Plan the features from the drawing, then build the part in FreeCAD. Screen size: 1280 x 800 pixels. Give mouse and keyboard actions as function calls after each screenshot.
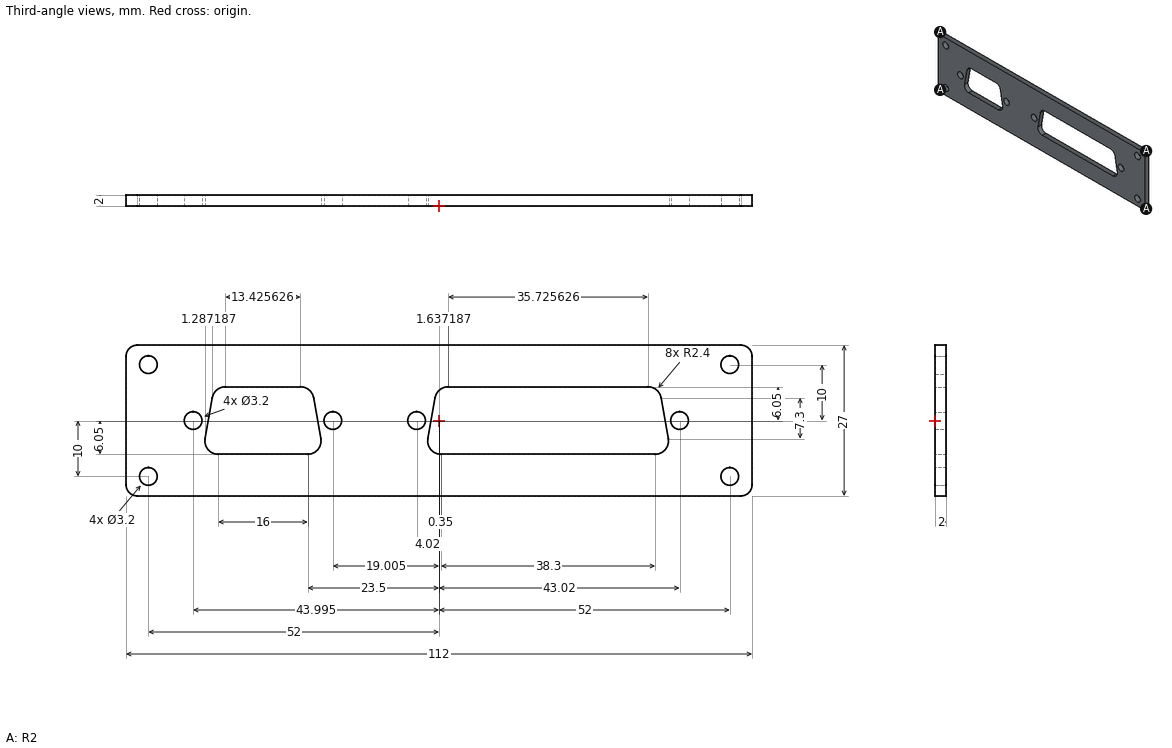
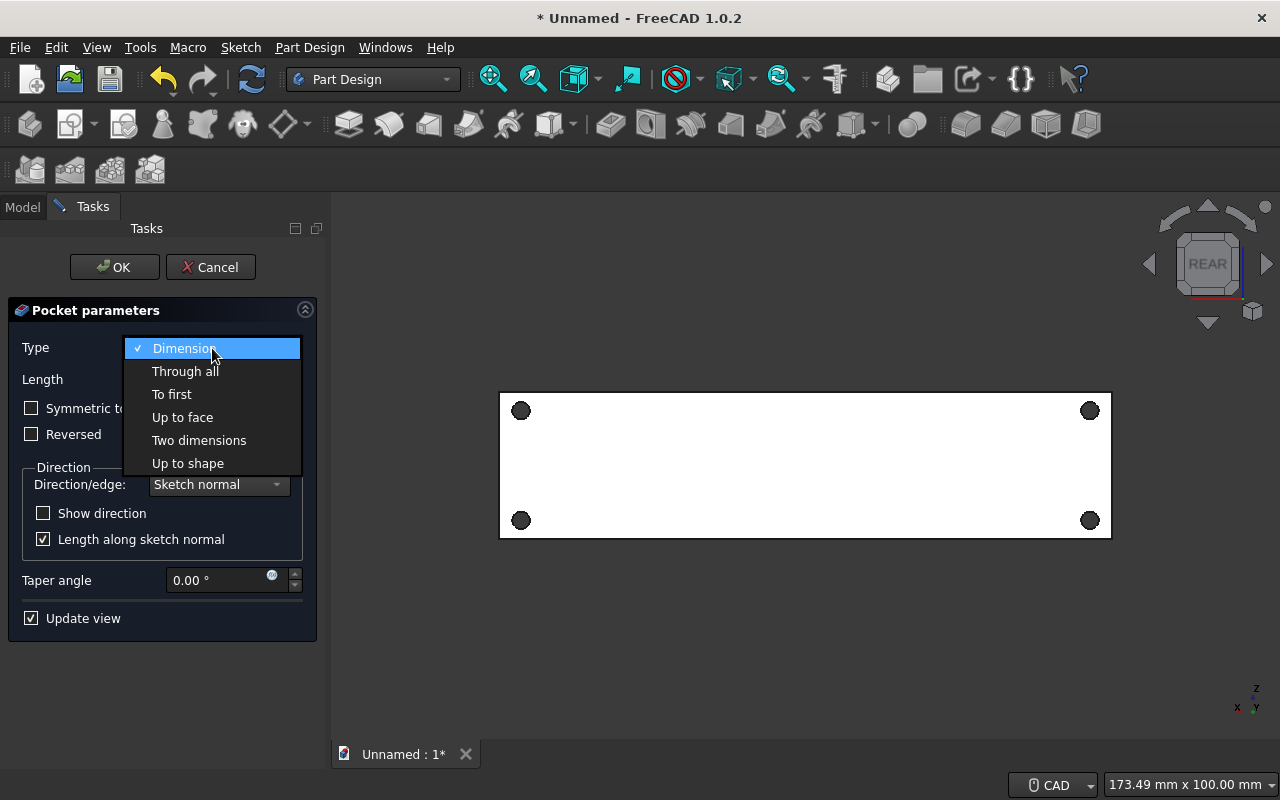
click(212, 372)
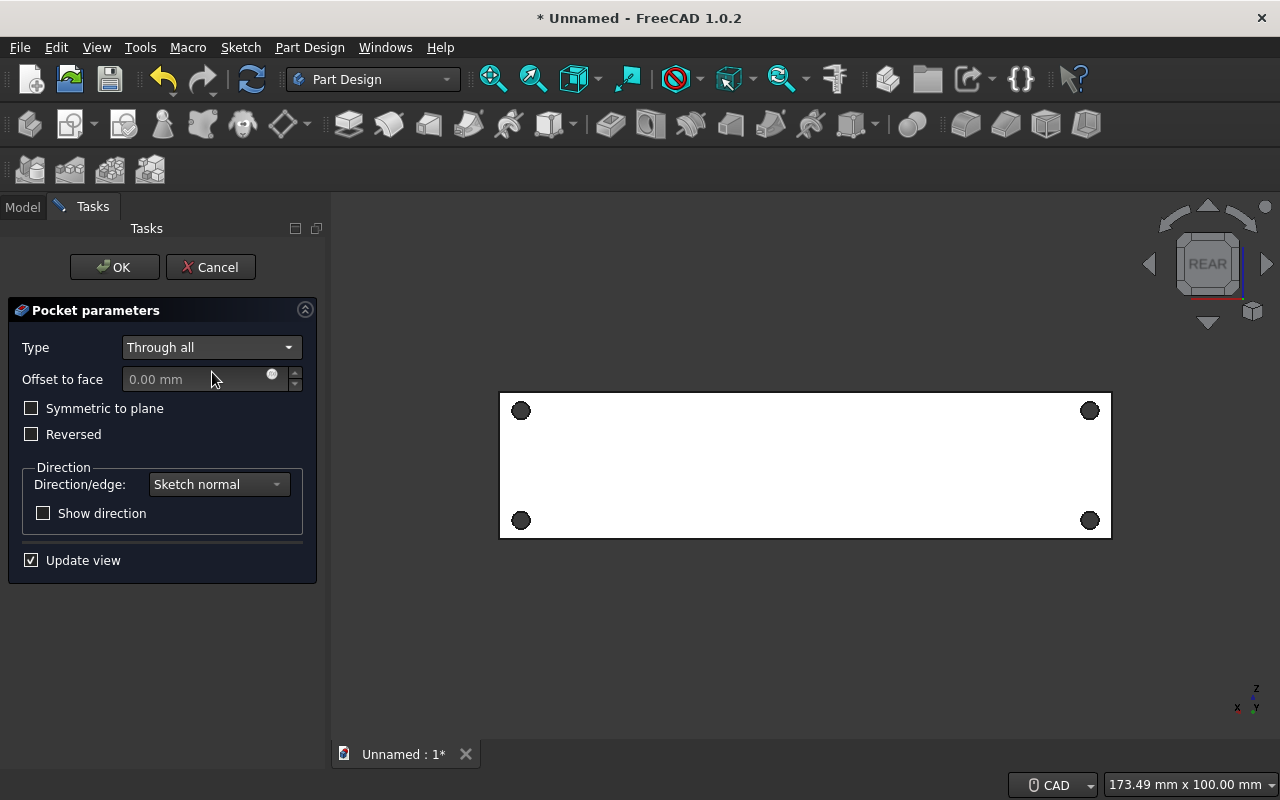
click(115, 267)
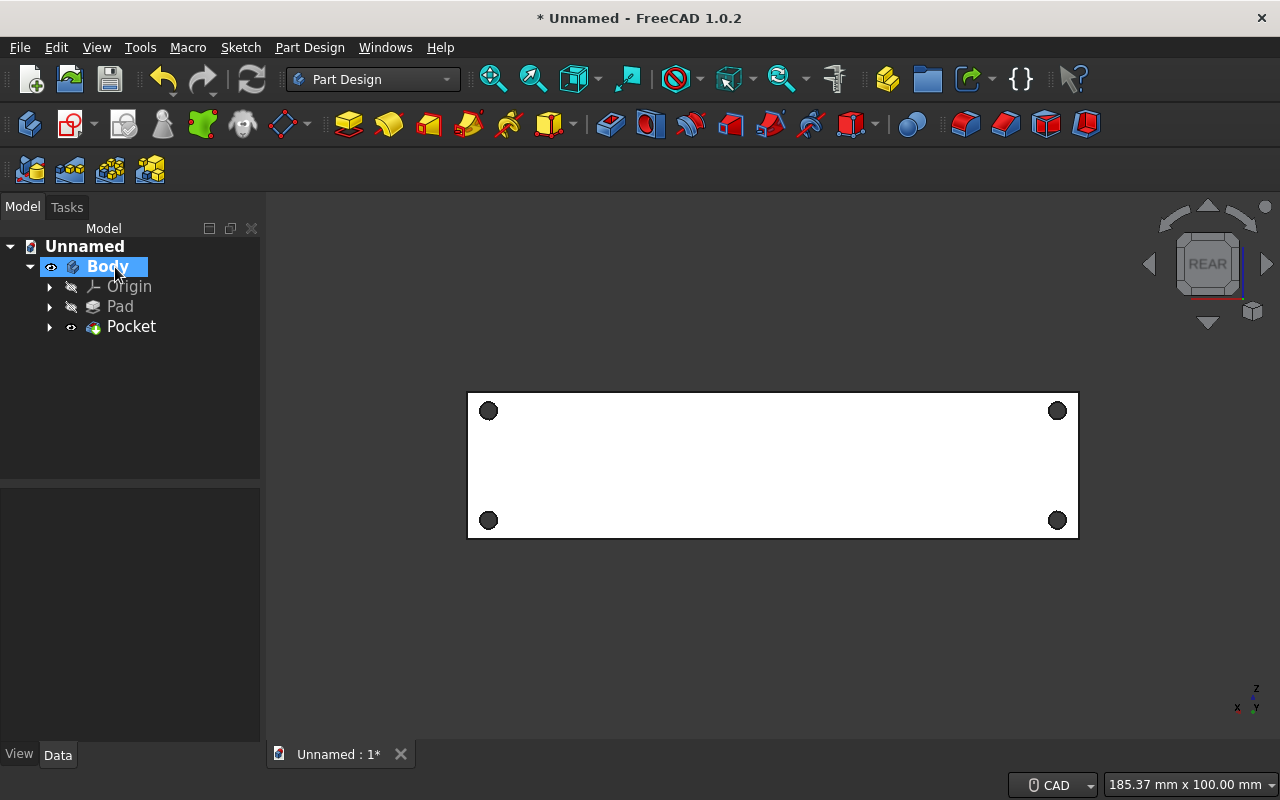
scroll(467, 391, up, 7)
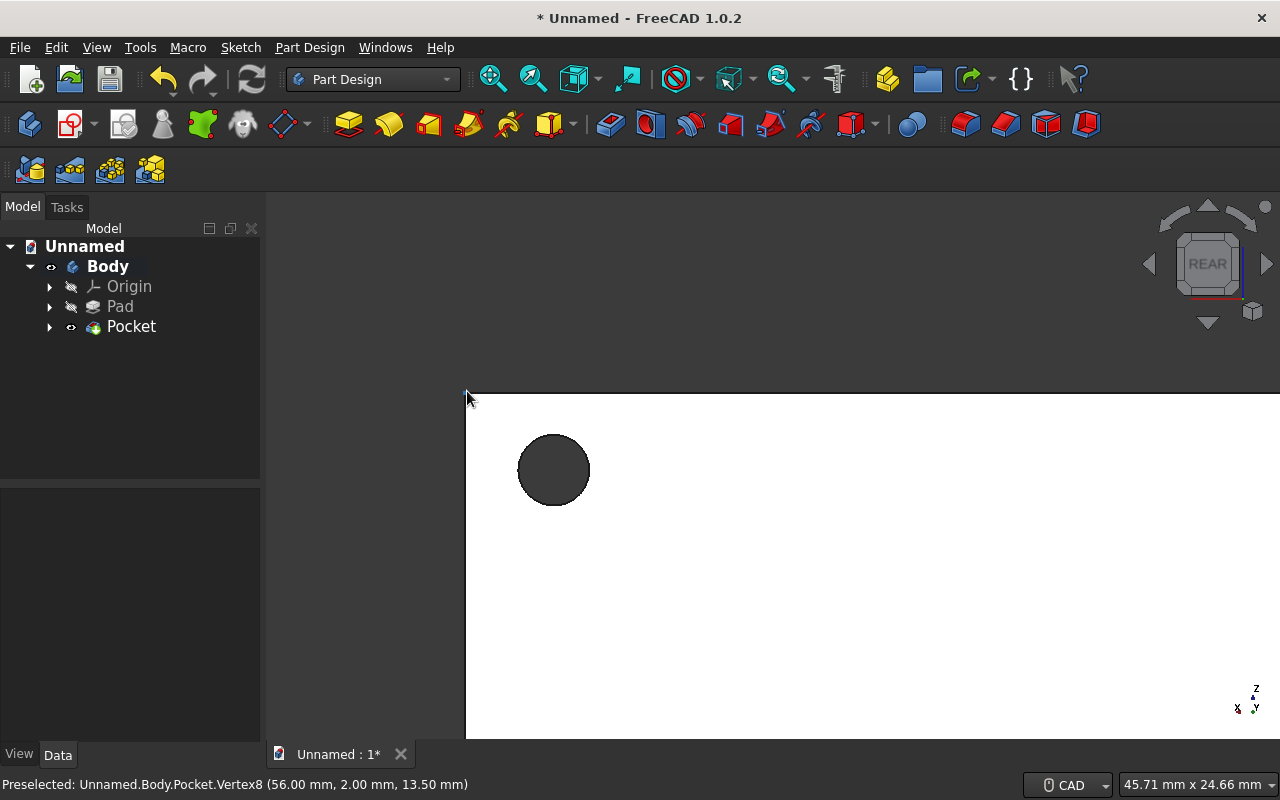
click(494, 80)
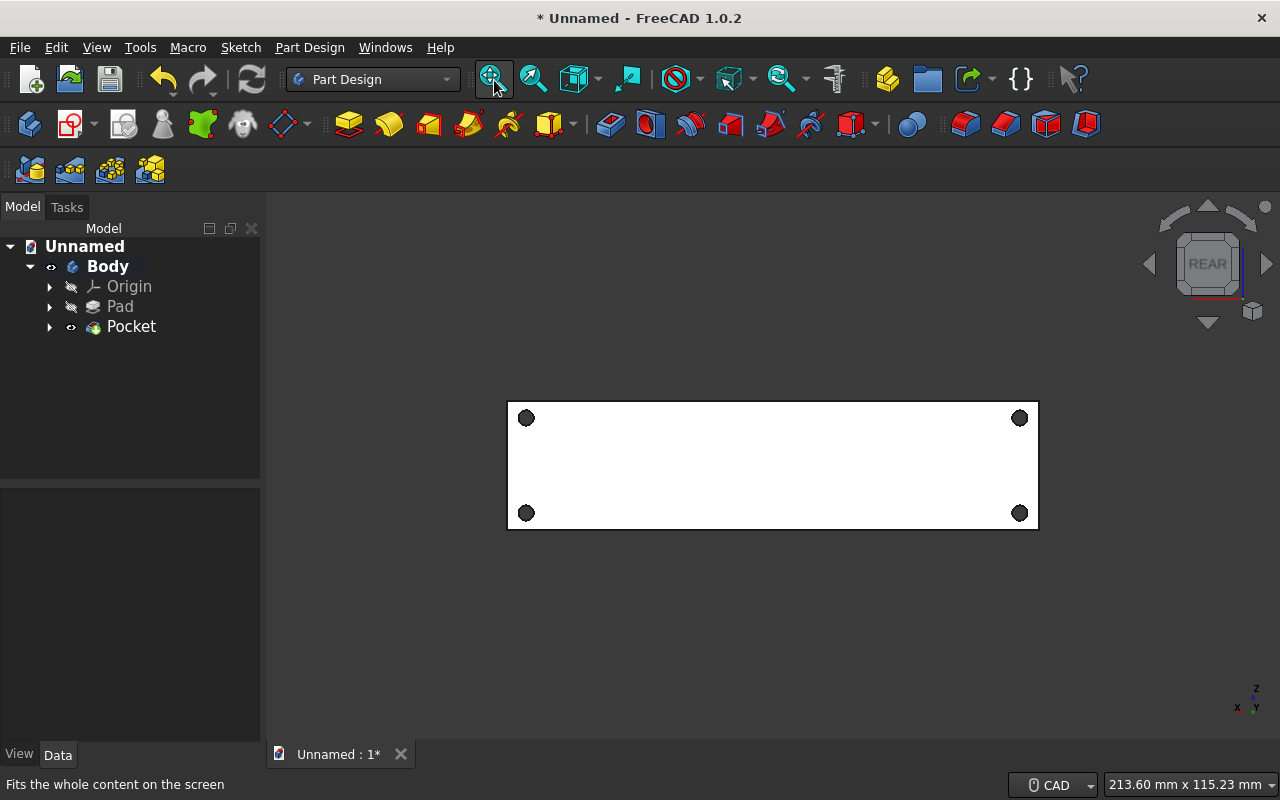
key(0)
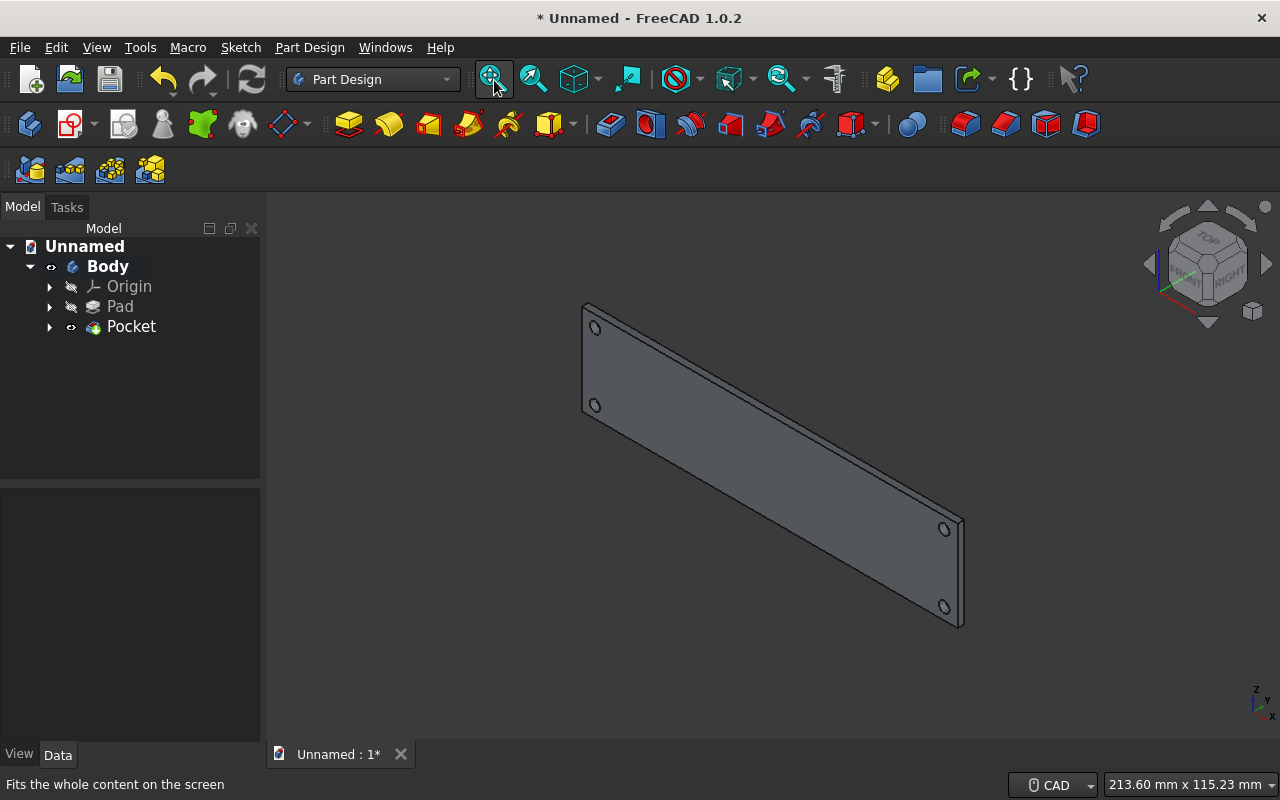
scroll(961, 521, up, 8)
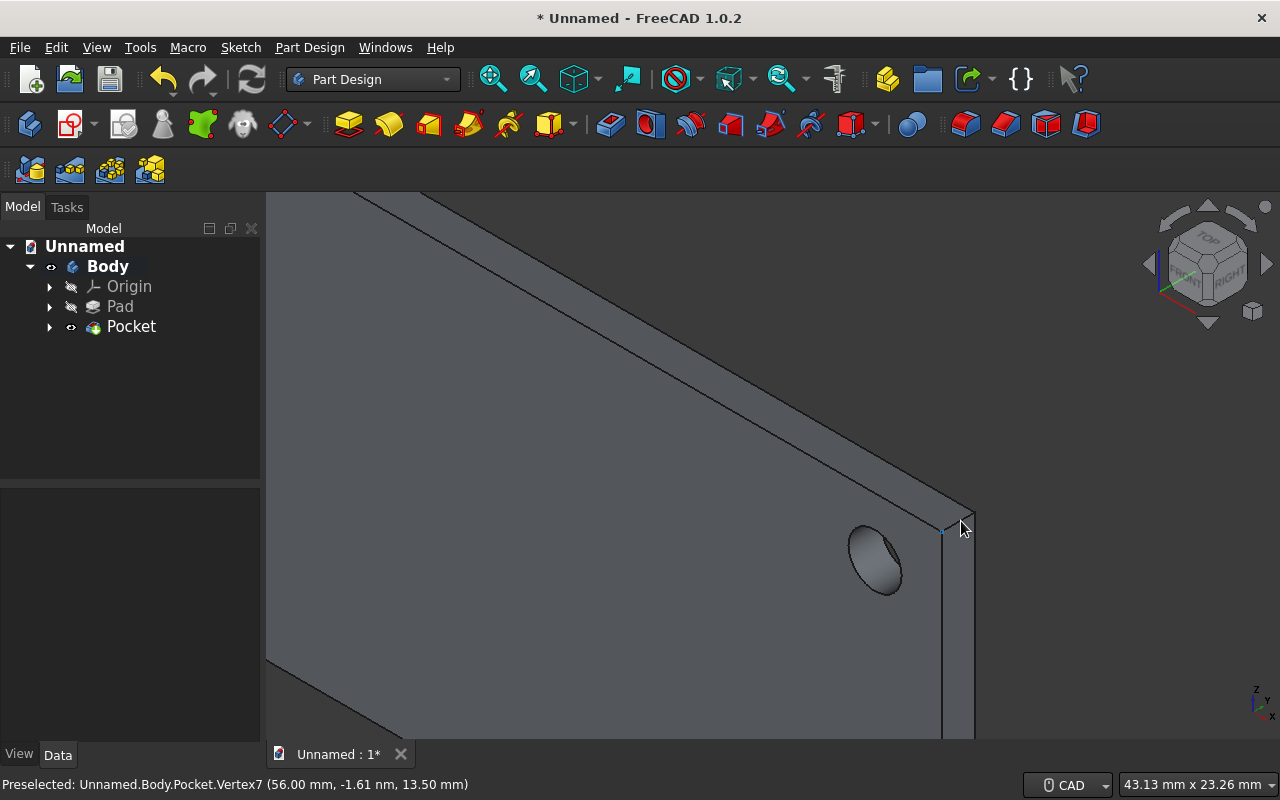
click(958, 521)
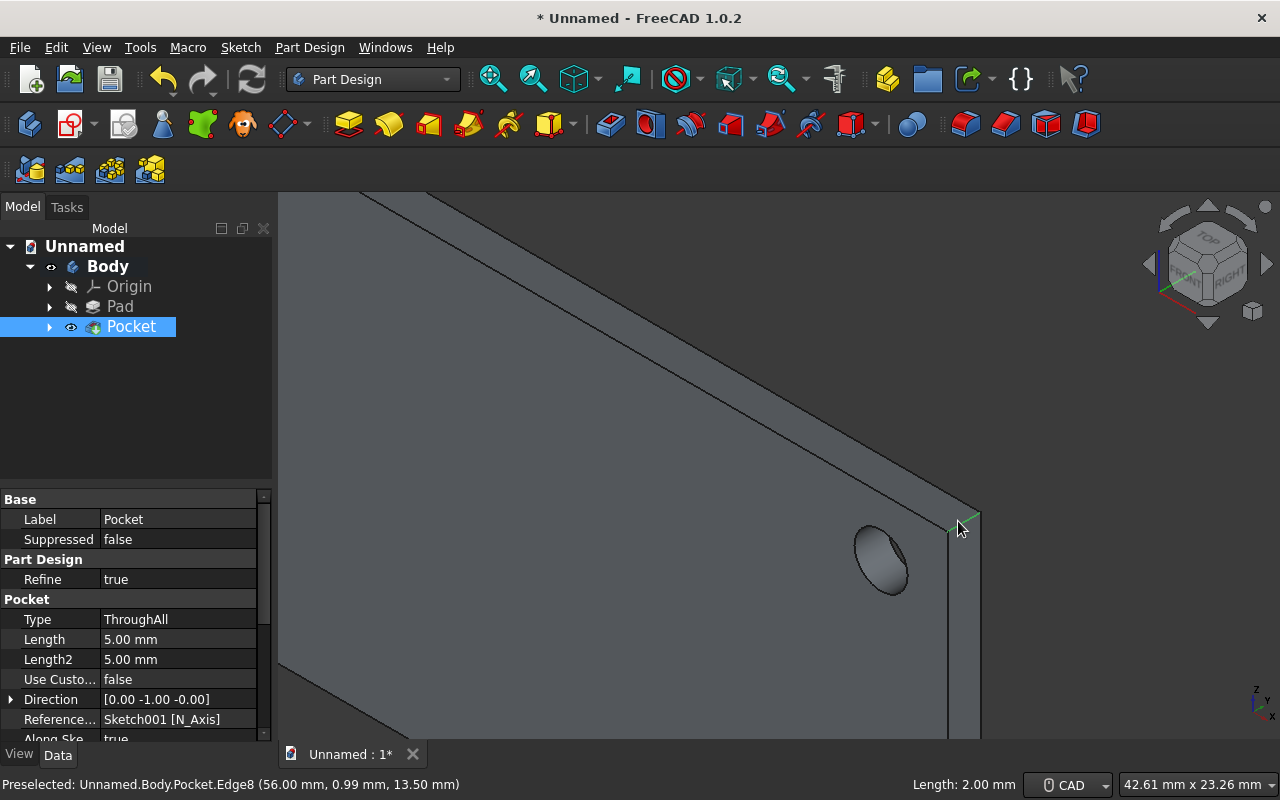
click(494, 80)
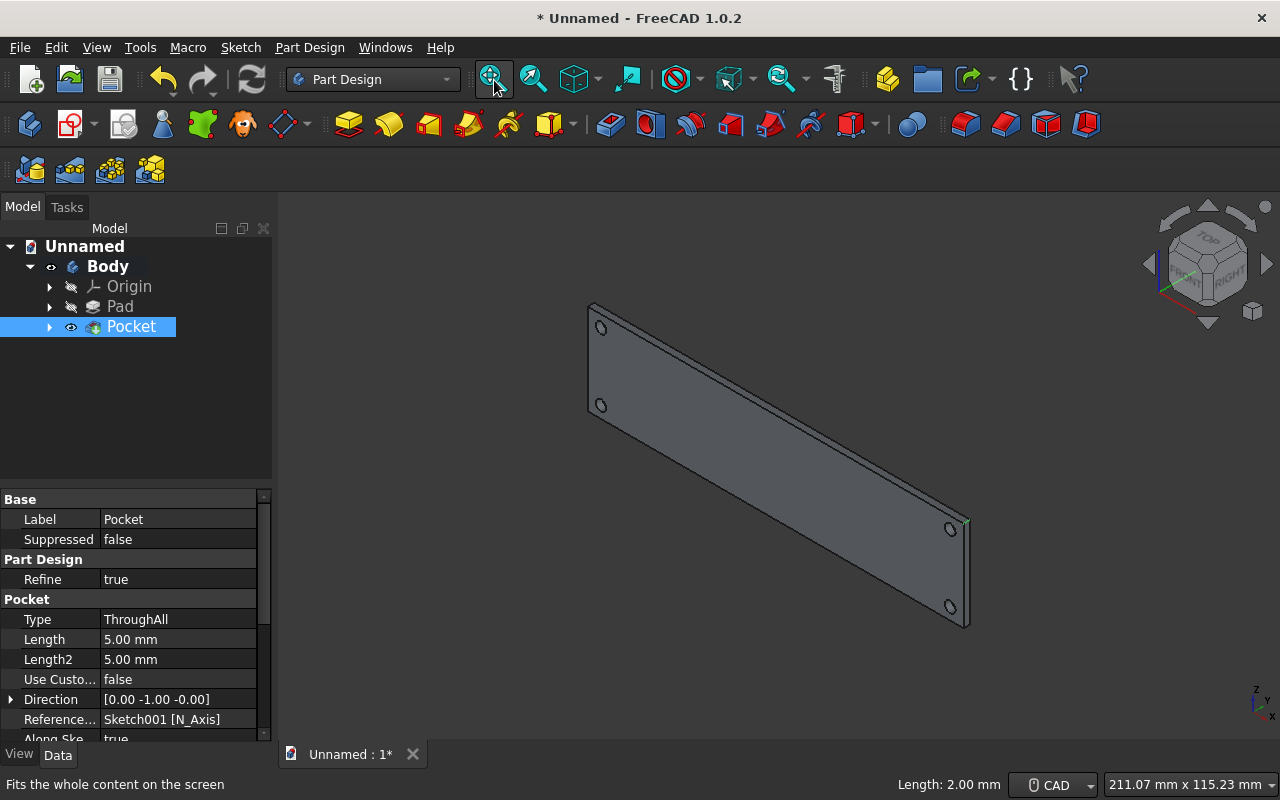
key(2)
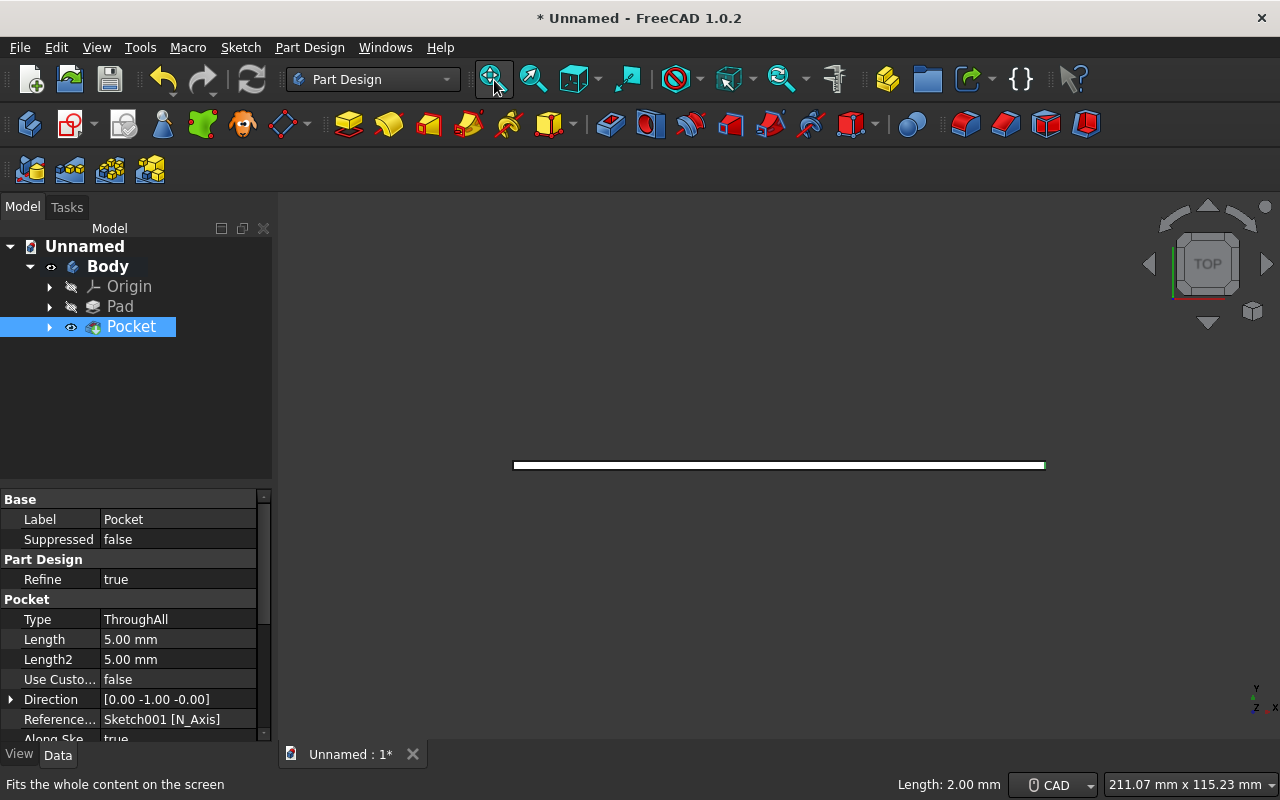
click(513, 466, ctrl)